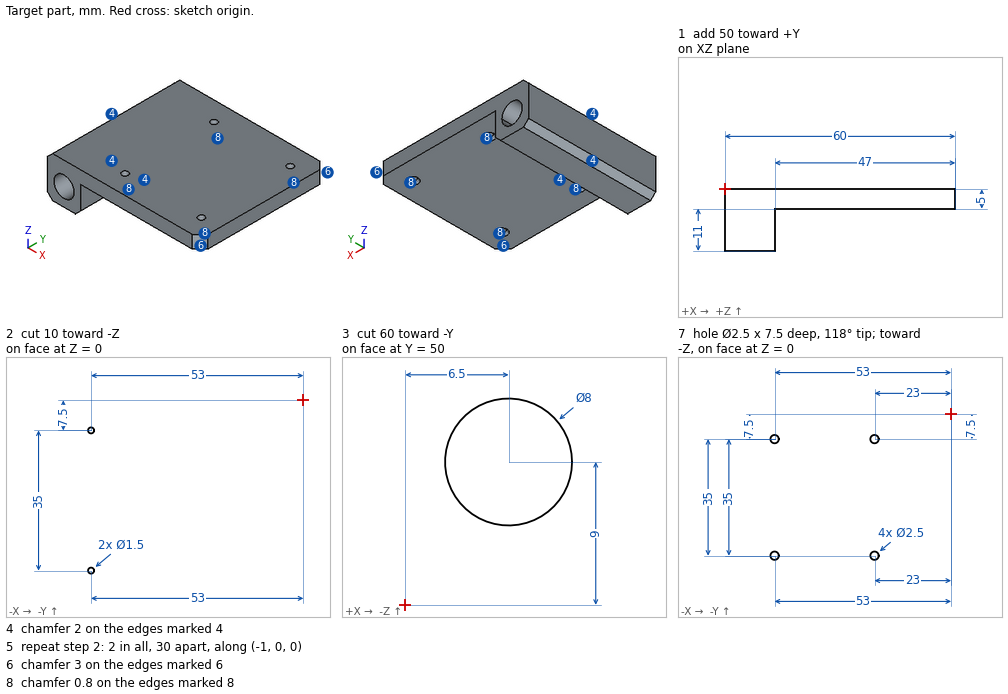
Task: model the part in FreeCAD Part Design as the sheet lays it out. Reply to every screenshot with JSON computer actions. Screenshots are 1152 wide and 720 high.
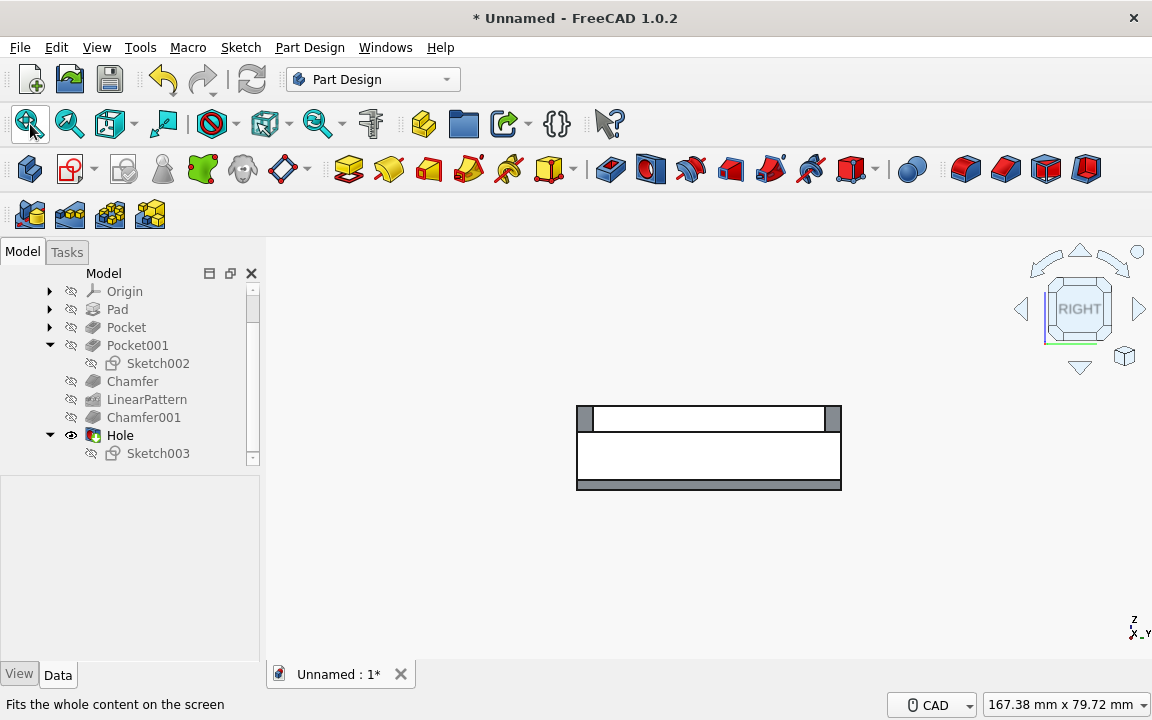
{"action": "key", "text": "5"}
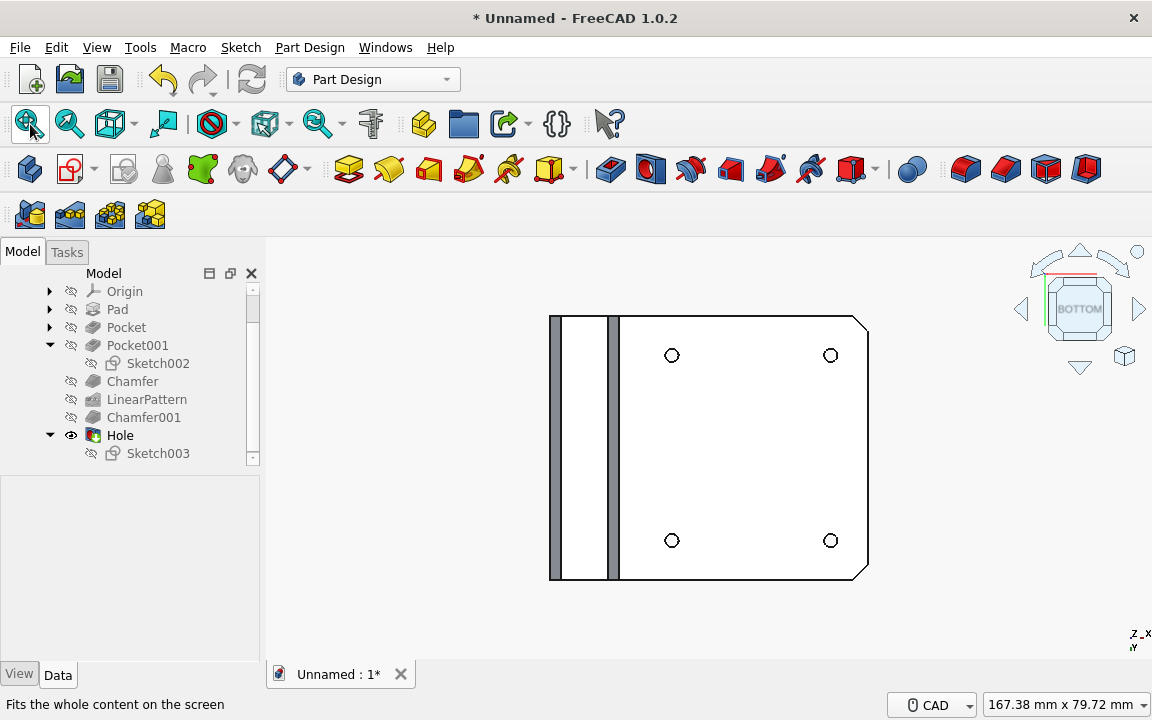
{"action": "left_click", "coordinate": [665, 354]}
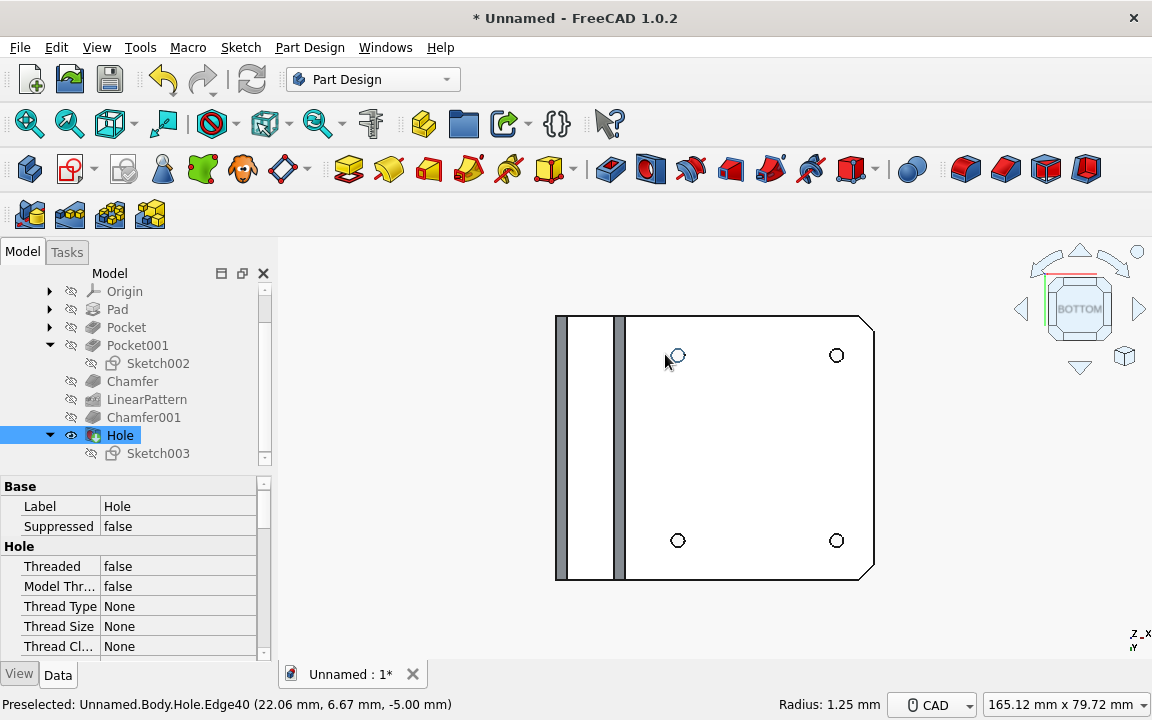
{"action": "left_click", "coordinate": [830, 354], "text": "ctrl"}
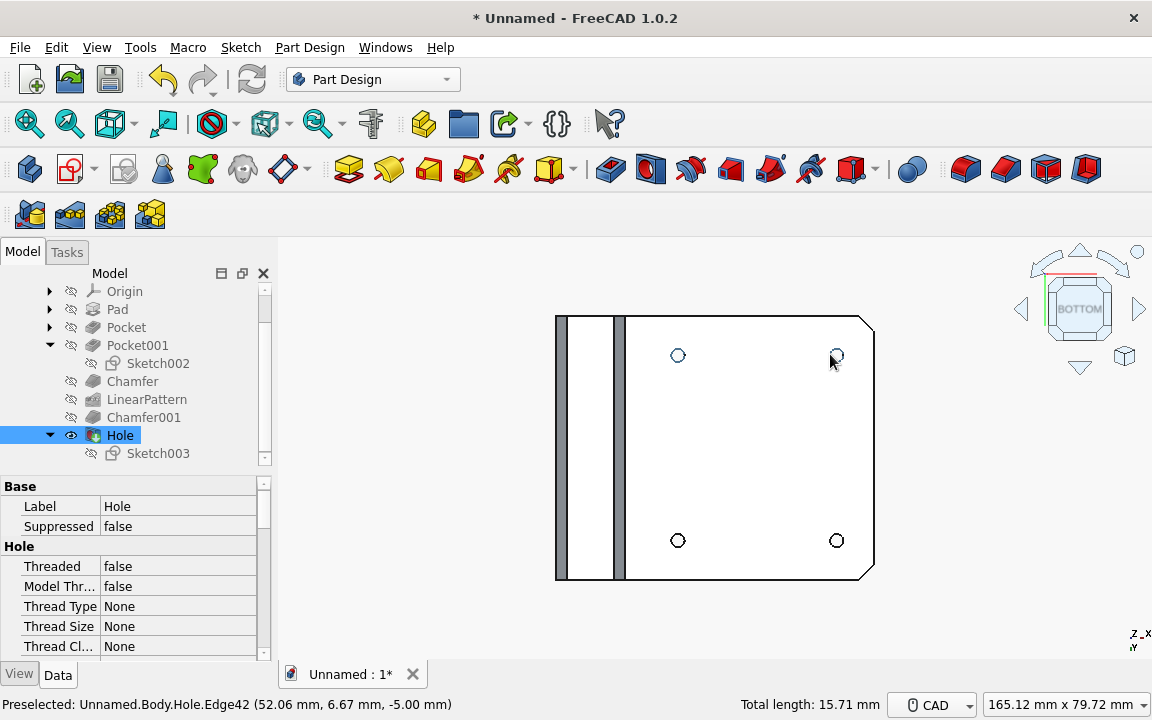
{"action": "left_click", "coordinate": [830, 540], "text": "ctrl"}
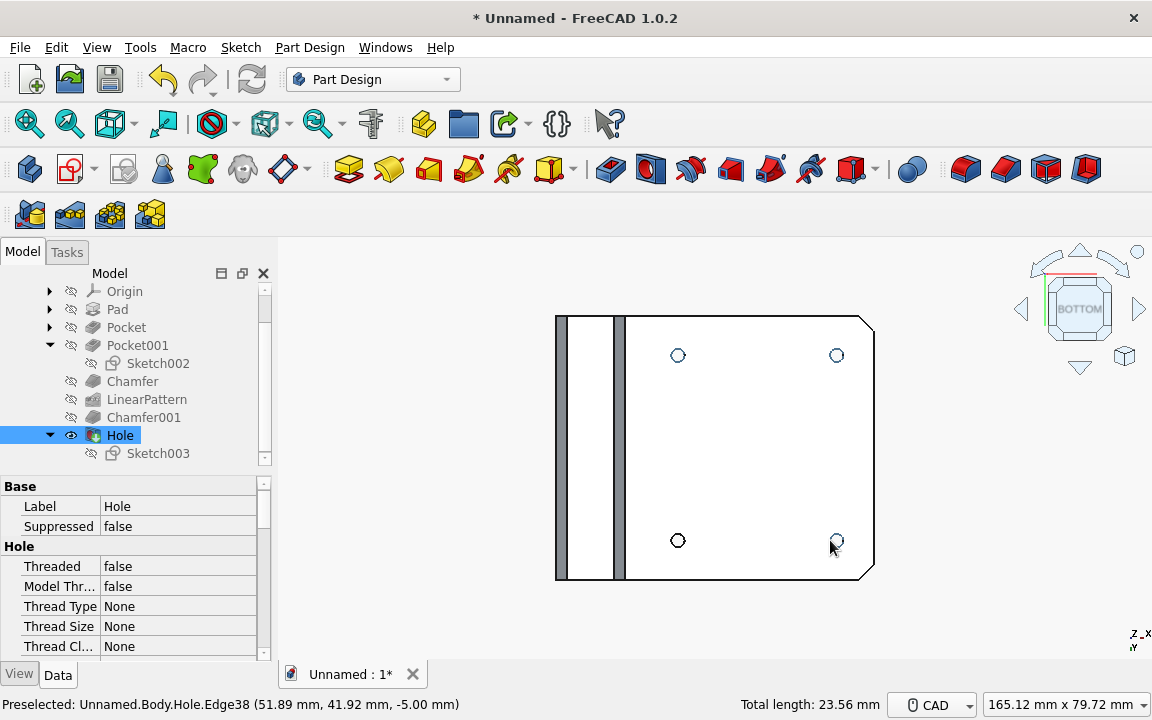
{"action": "left_click", "coordinate": [671, 540], "text": "ctrl"}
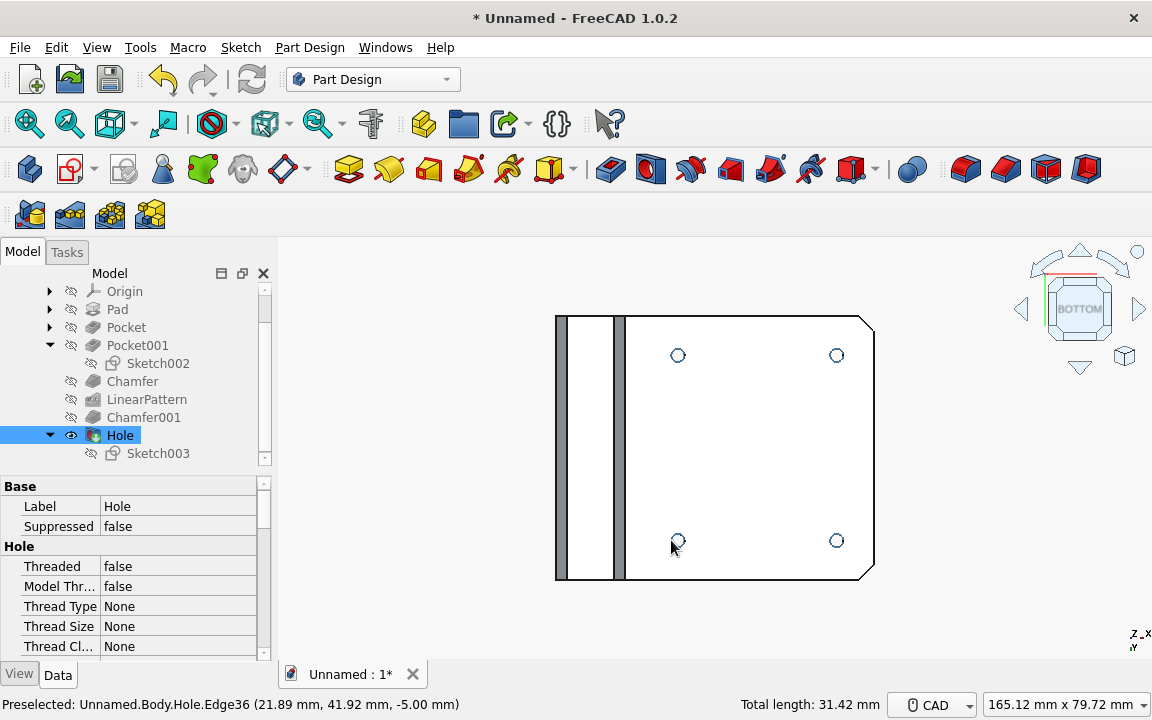
{"action": "left_click", "coordinate": [1006, 170]}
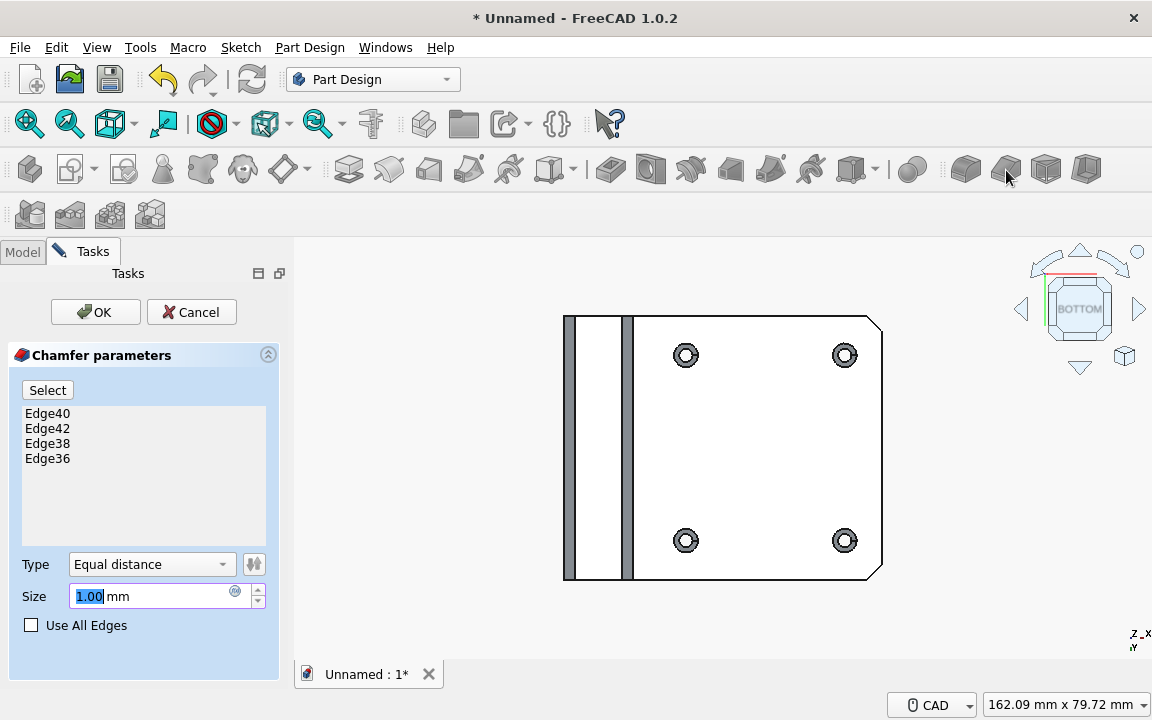
{"action": "type", "text": "0.8"}
{"action": "key", "text": "Tab"}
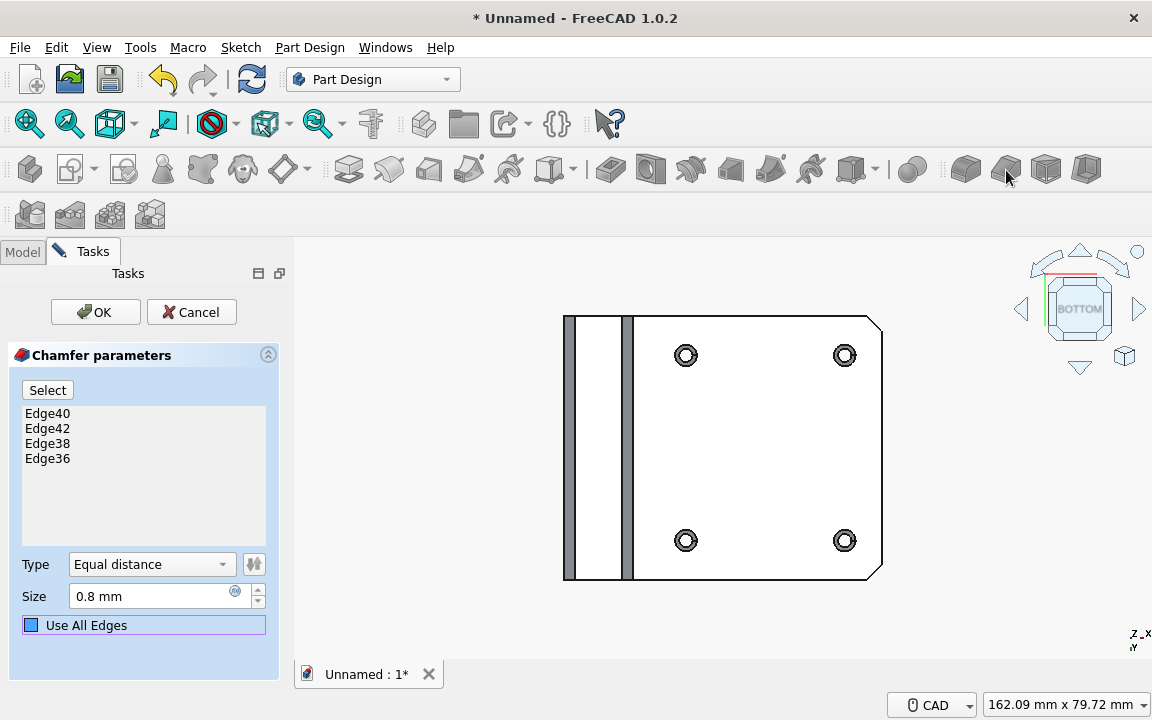
{"action": "left_click", "coordinate": [96, 312]}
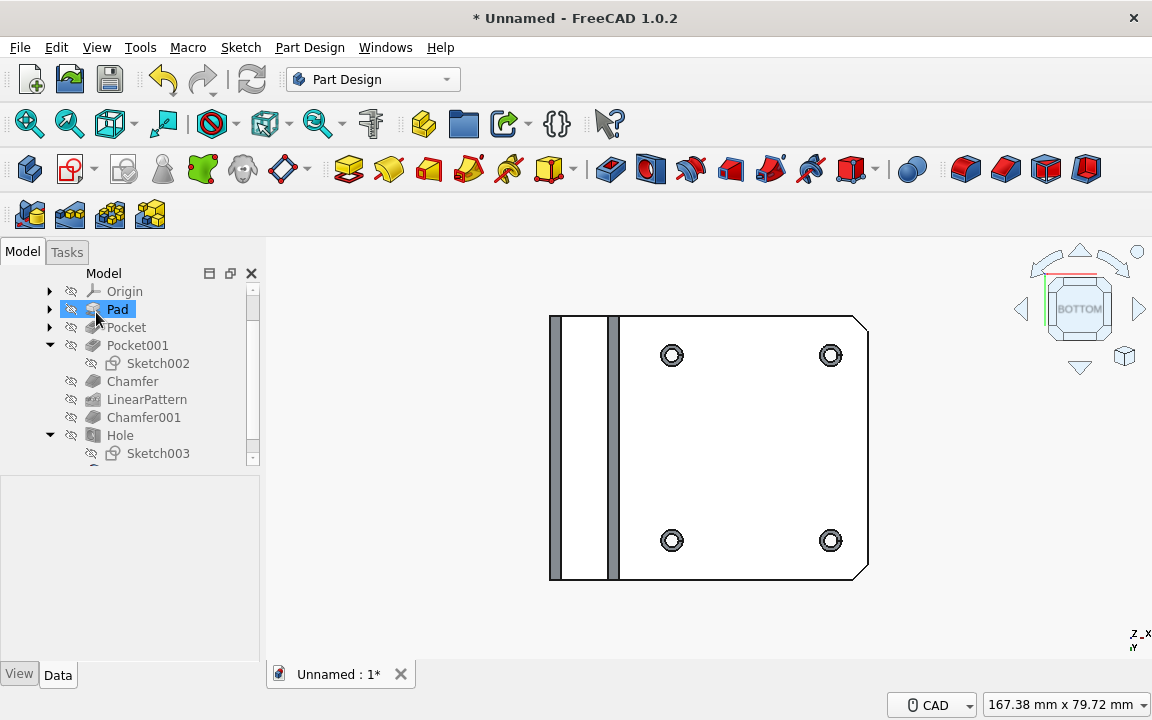
{"action": "key", "text": "0"}